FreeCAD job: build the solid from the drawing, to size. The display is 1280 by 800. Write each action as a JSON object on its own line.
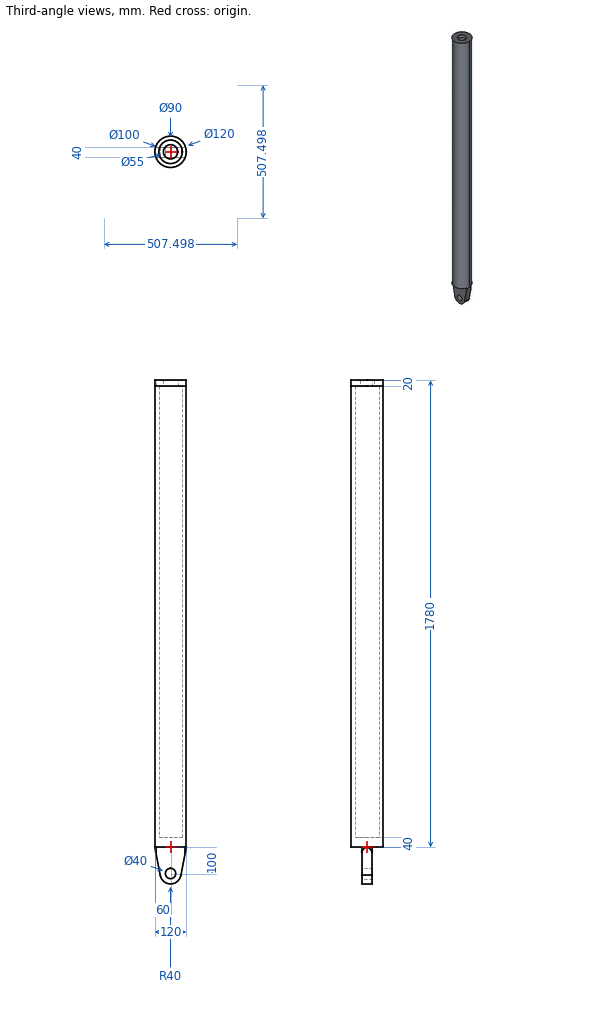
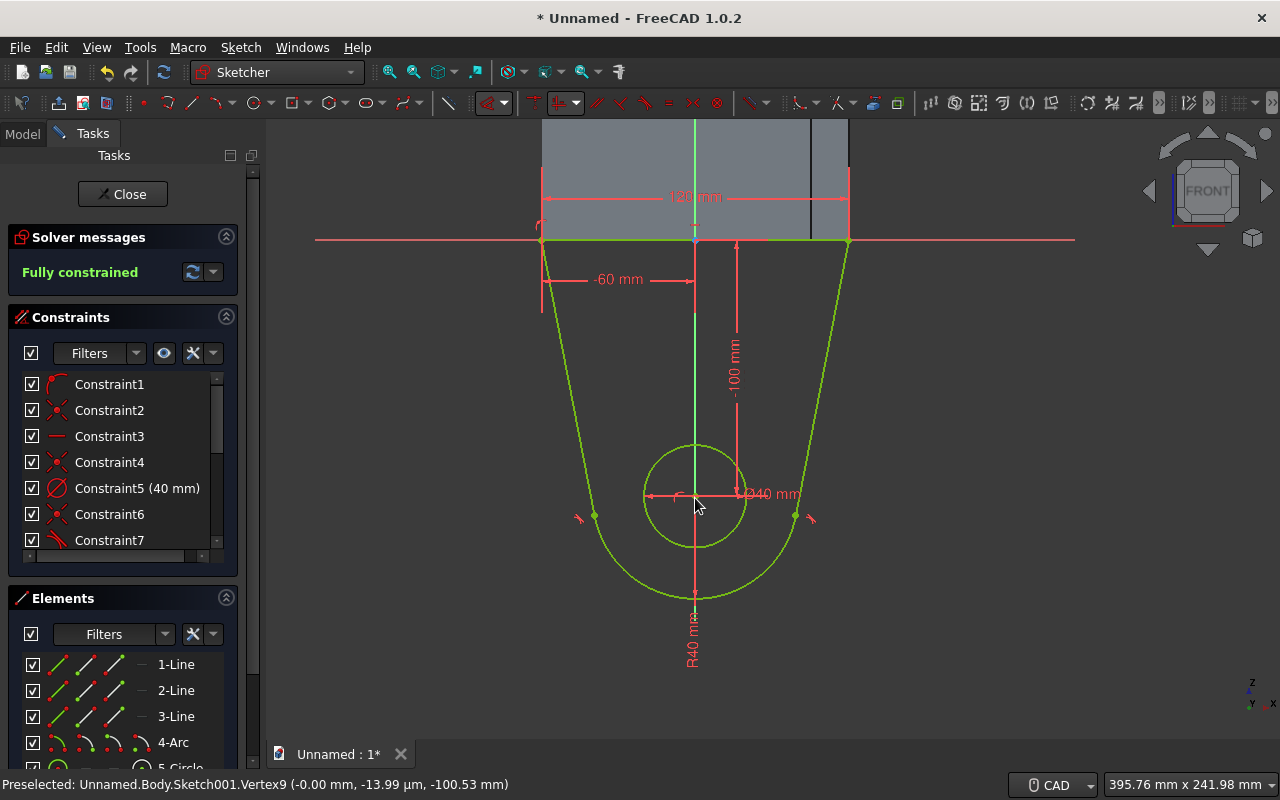
{"action": "left_click", "coordinate": [123, 194]}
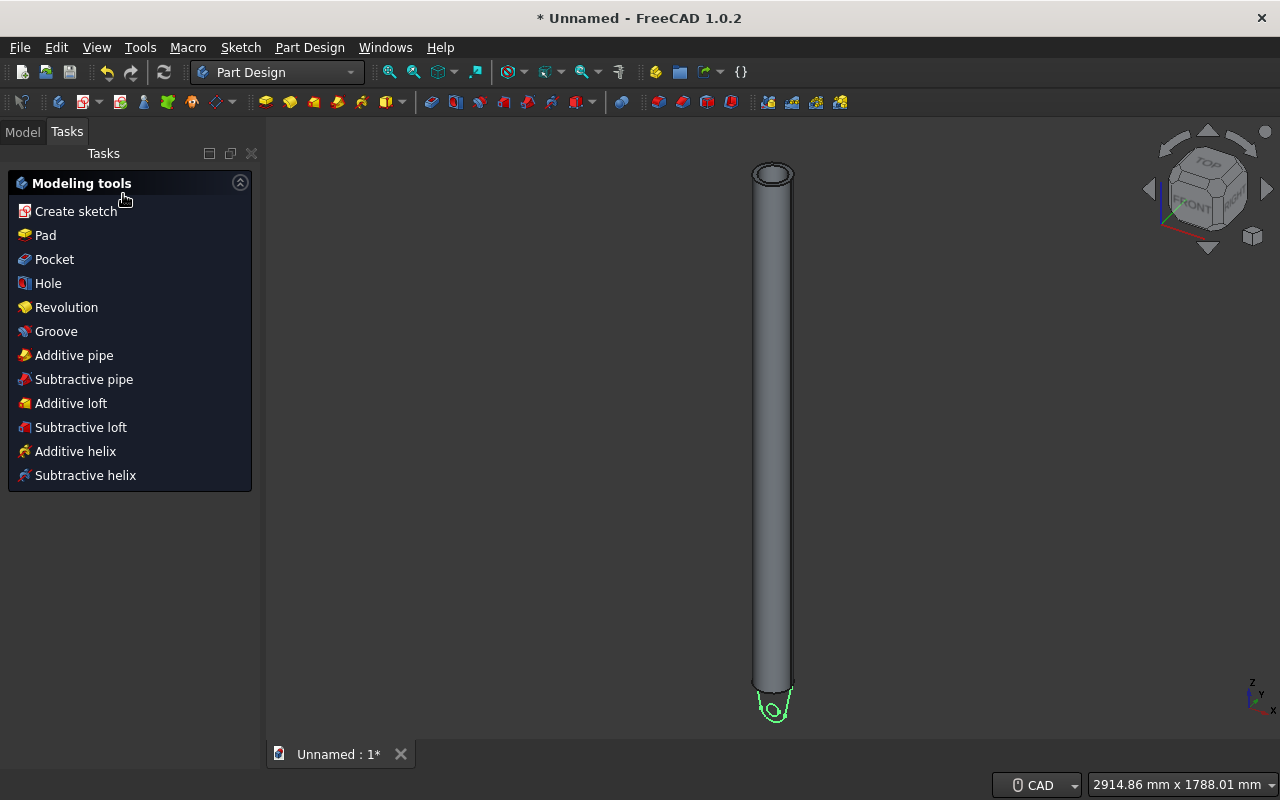
{"action": "left_click", "coordinate": [266, 102]}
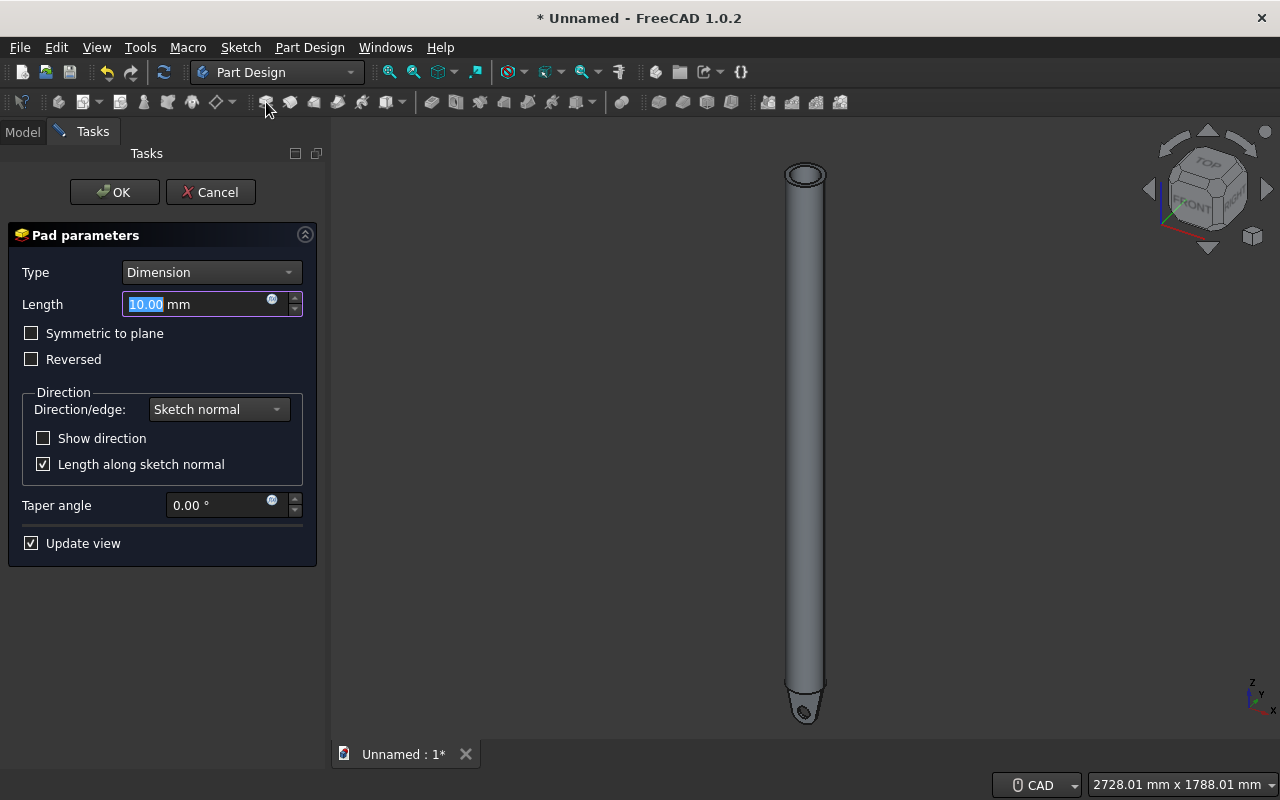
{"action": "type", "text": "40"}
{"action": "key", "text": "Tab"}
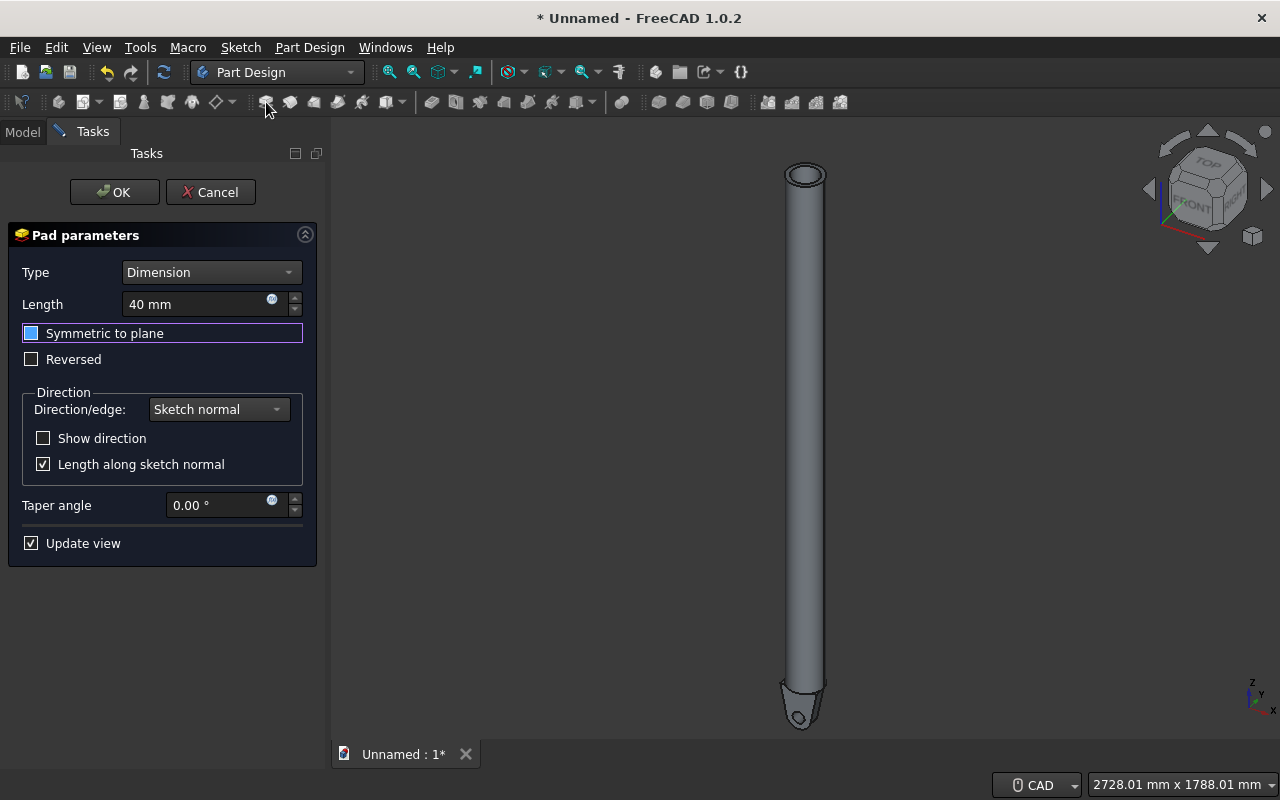
{"action": "left_click", "coordinate": [30, 333]}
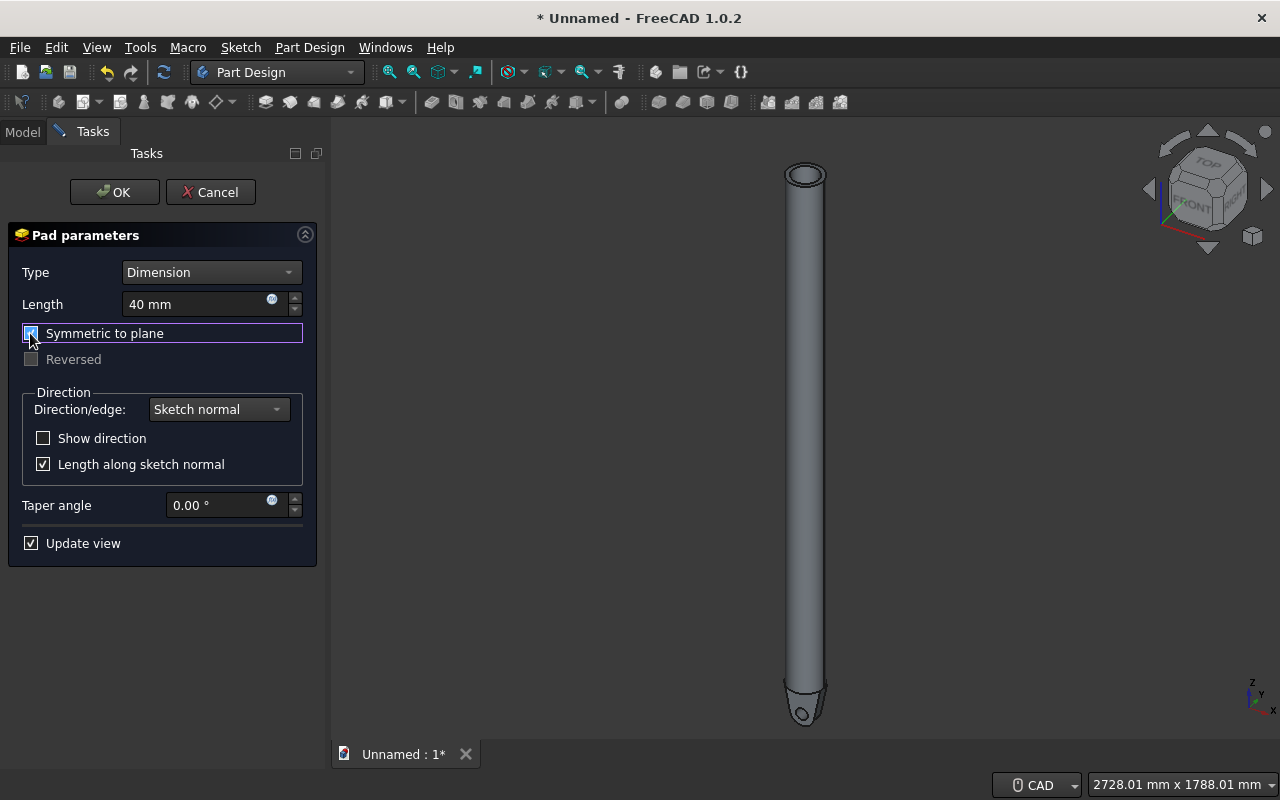
{"action": "left_click", "coordinate": [115, 192]}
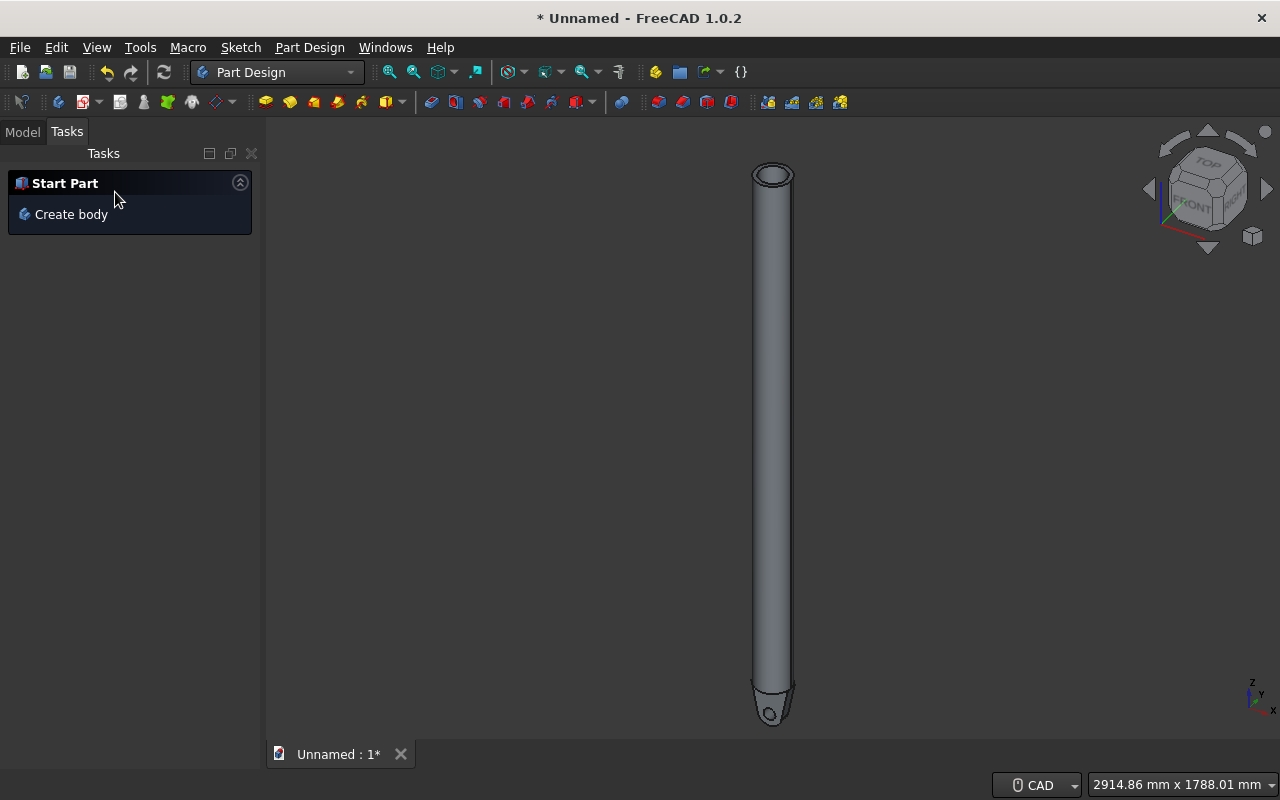
{"action": "left_click", "coordinate": [84, 102]}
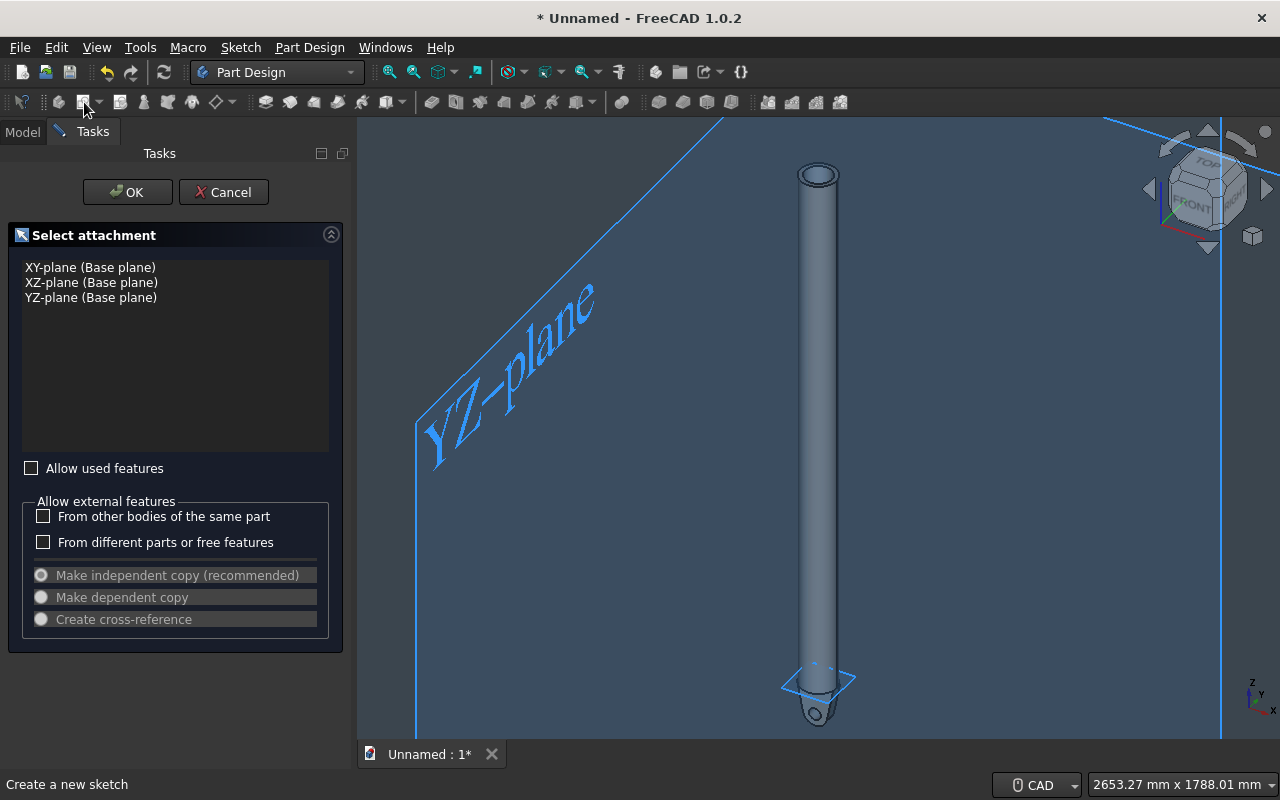
{"action": "left_click", "coordinate": [82, 268]}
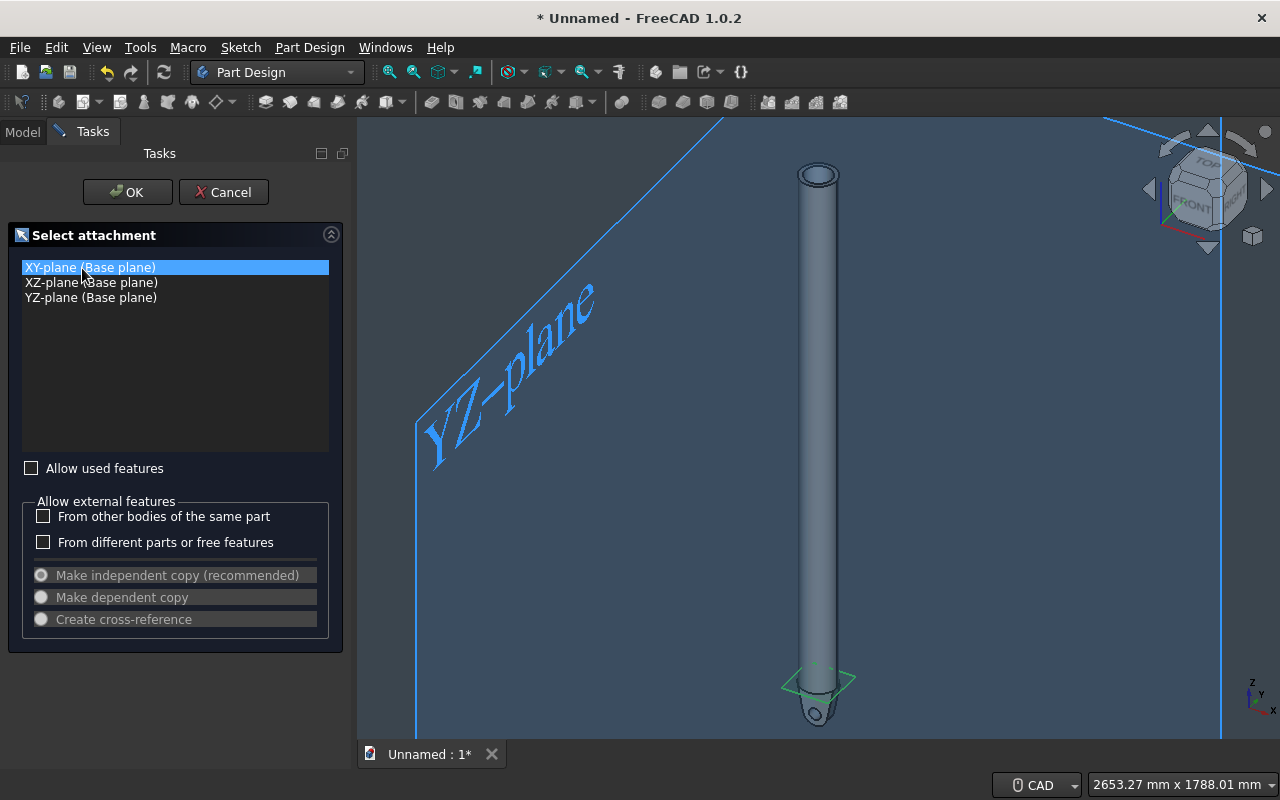
{"action": "left_click", "coordinate": [128, 192]}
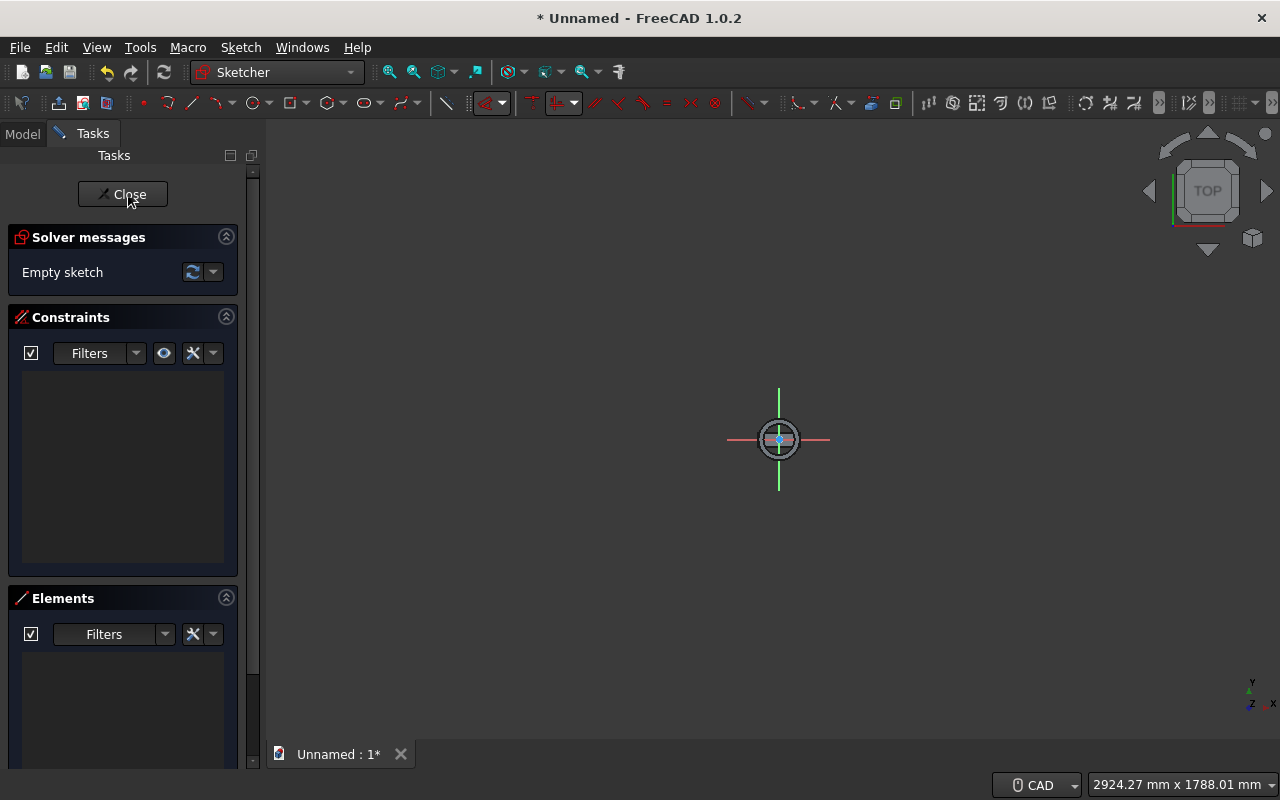
{"action": "key", "text": "q s"}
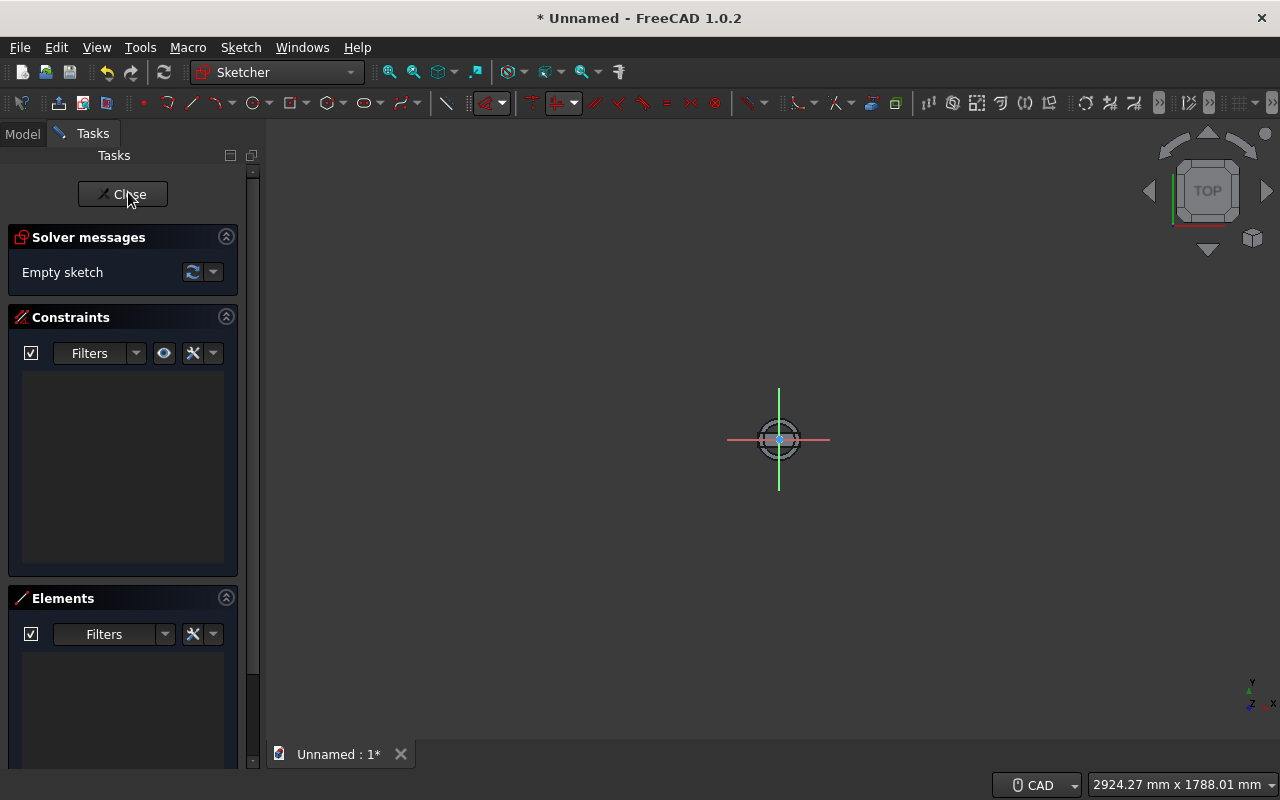
{"action": "scroll", "coordinate": [787, 441], "scroll_direction": "up", "scroll_amount": 12}